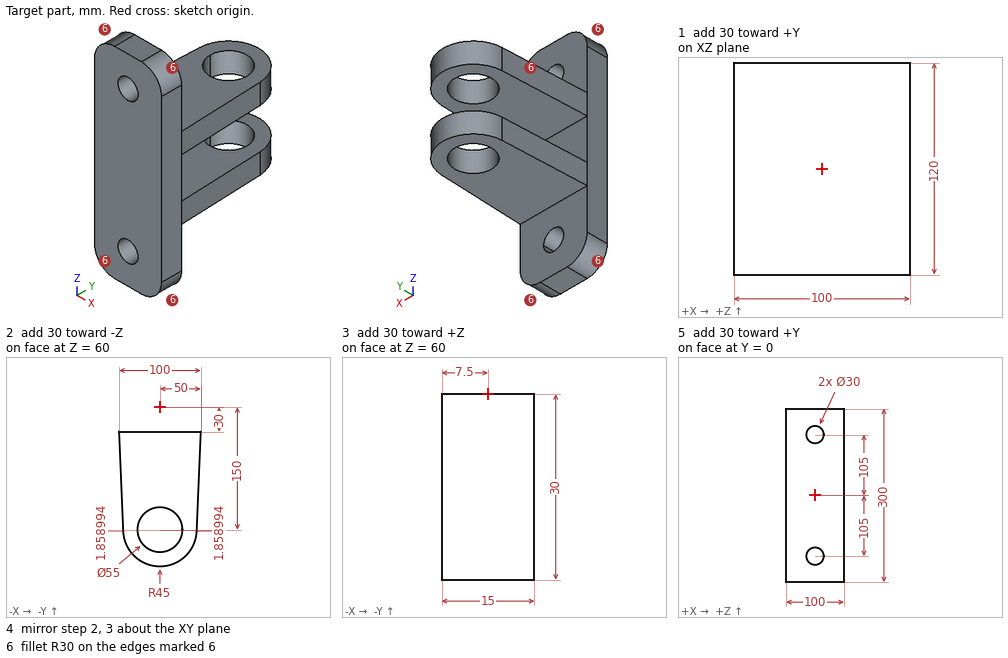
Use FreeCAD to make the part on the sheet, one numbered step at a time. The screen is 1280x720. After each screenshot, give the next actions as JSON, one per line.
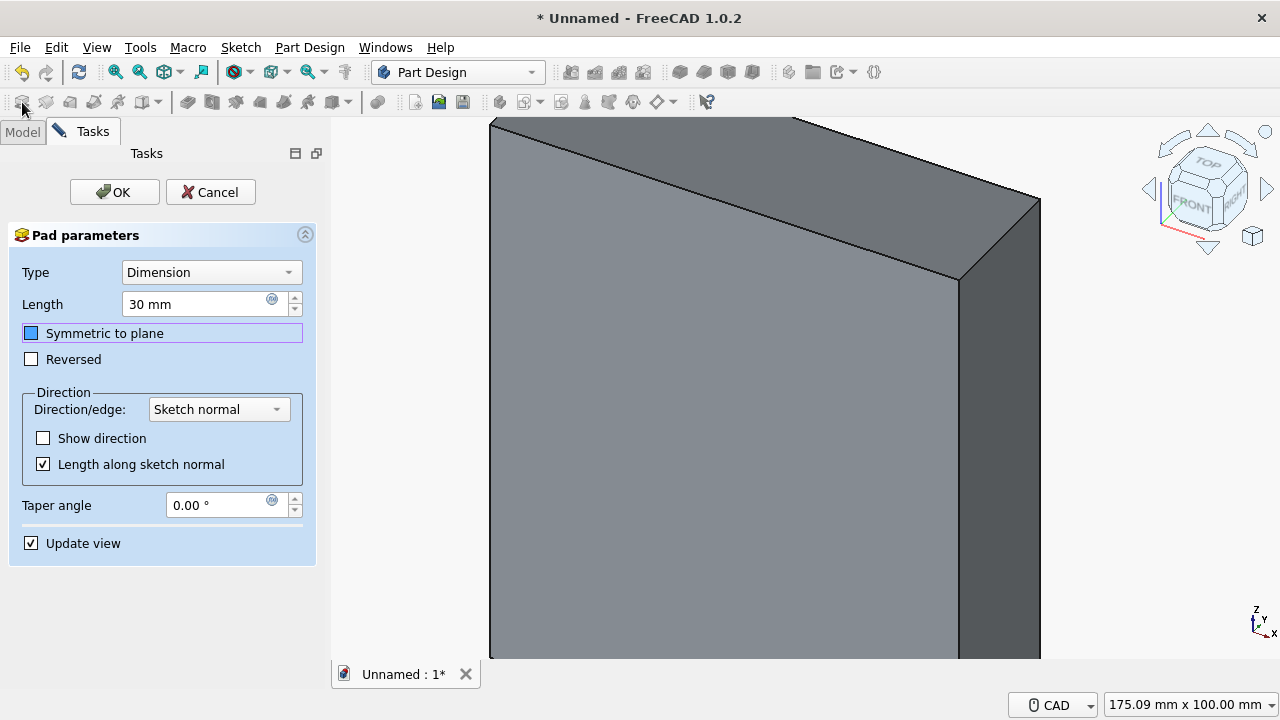
{"action": "left_click", "coordinate": [30, 359]}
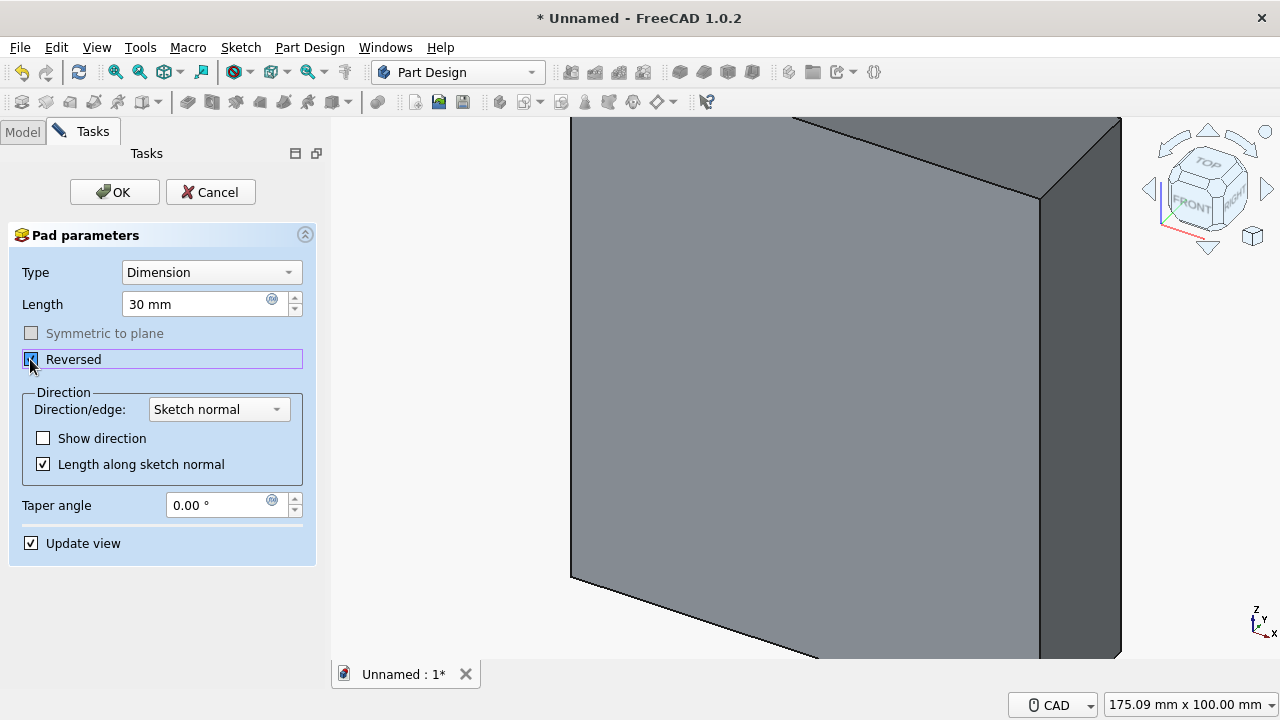
{"action": "left_click", "coordinate": [115, 192]}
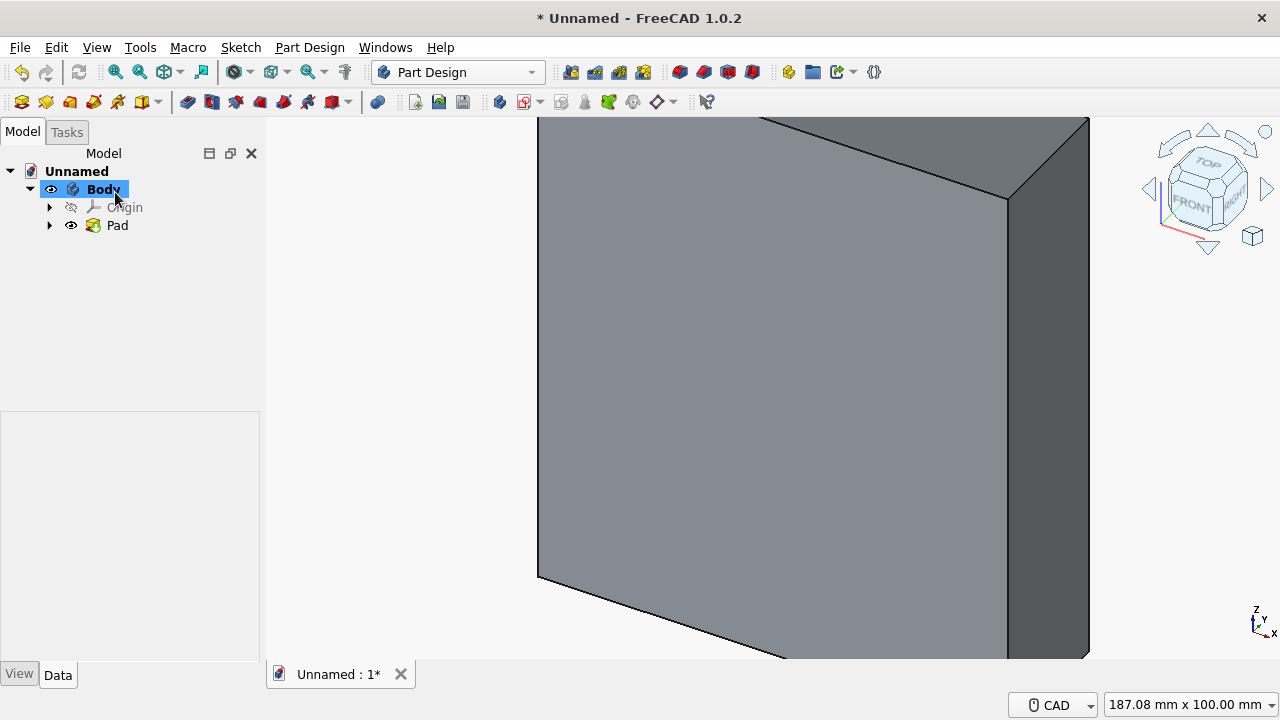
{"action": "key", "text": "v f"}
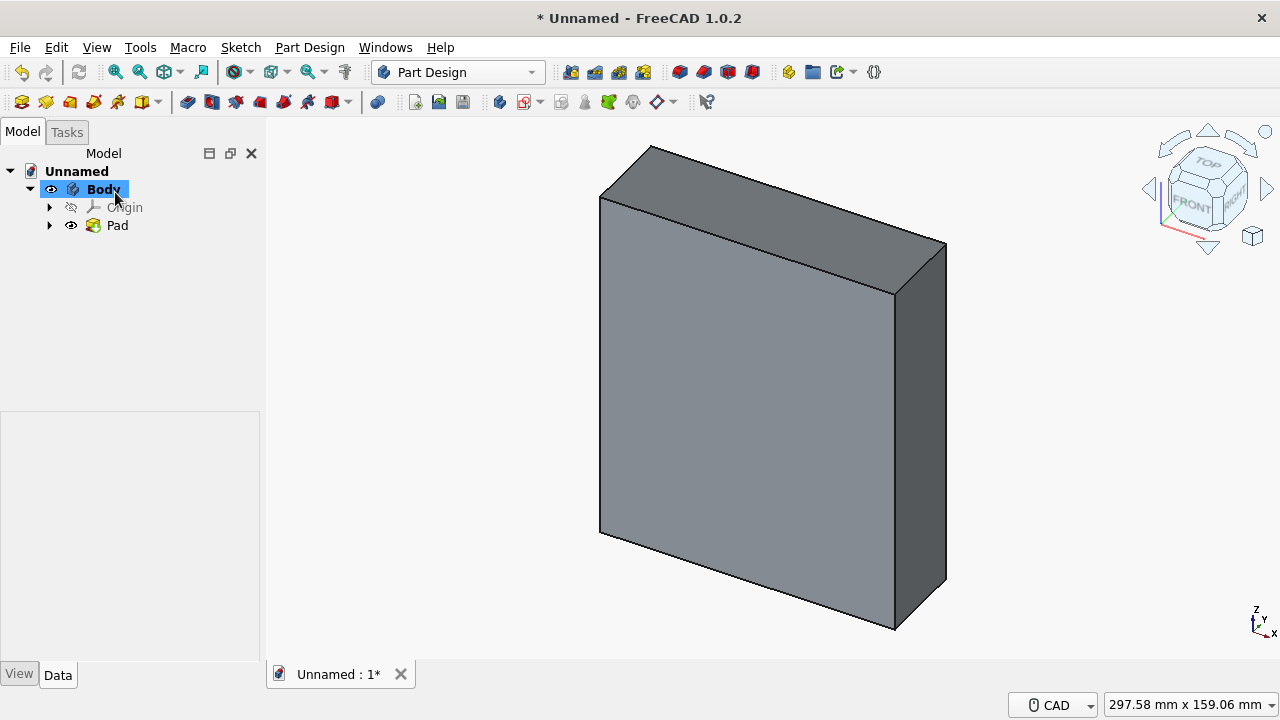
{"action": "left_click", "coordinate": [857, 247]}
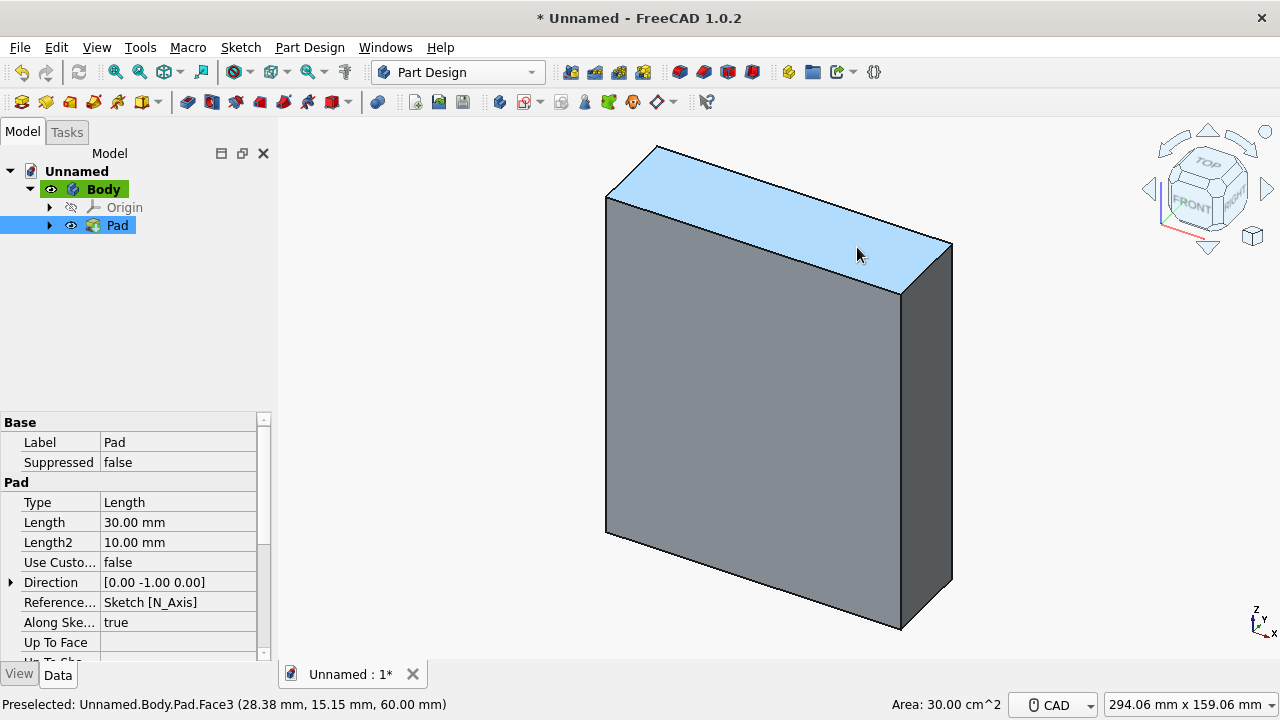
{"action": "left_click", "coordinate": [524, 102]}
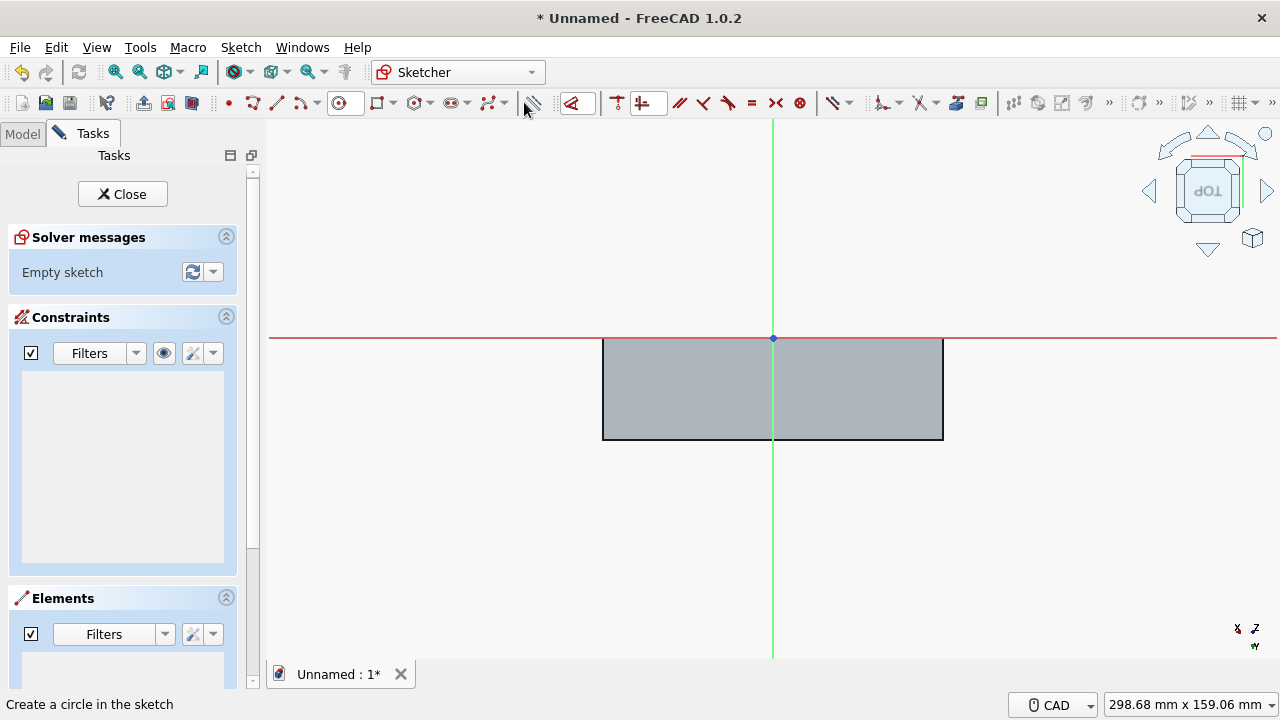
{"action": "scroll", "coordinate": [649, 160], "scroll_direction": "down", "scroll_amount": 4}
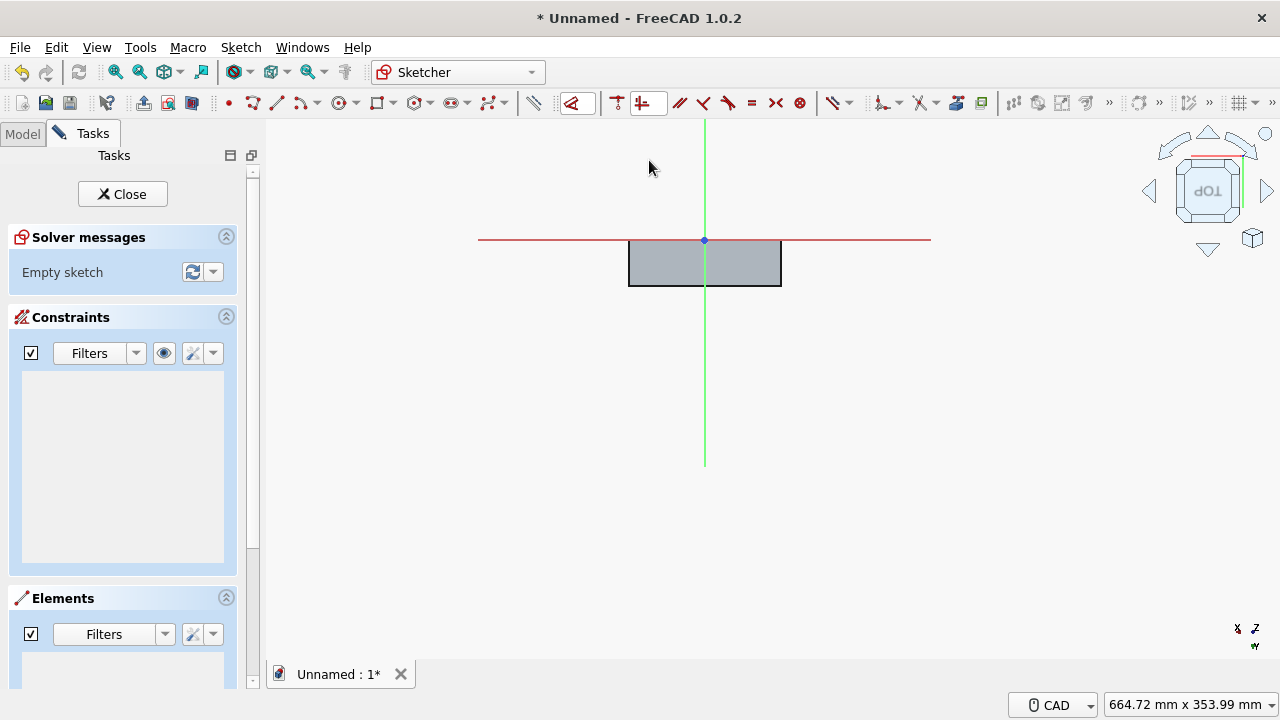
{"action": "key", "text": "g m"}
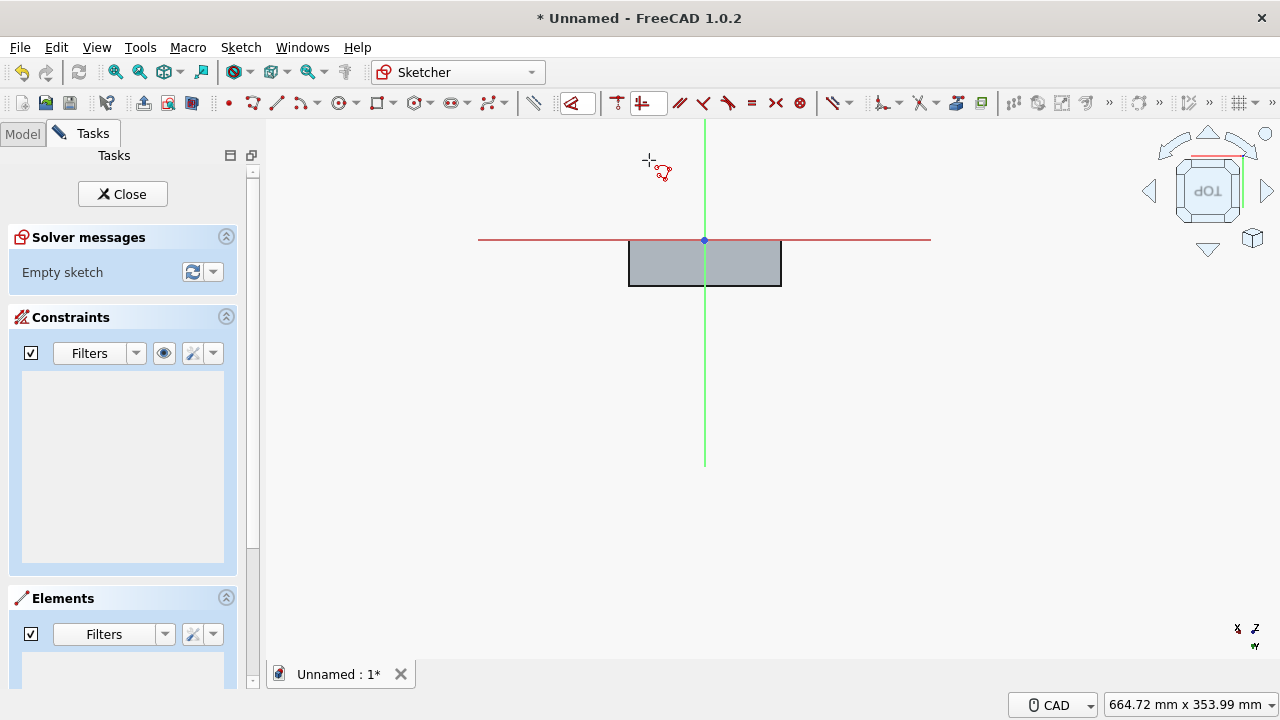
{"action": "left_click", "coordinate": [774, 472]}
{"action": "left_click", "coordinate": [784, 286]}
{"action": "left_click", "coordinate": [629, 286]}
{"action": "left_click", "coordinate": [639, 472]}
{"action": "right_click", "coordinate": [639, 472]}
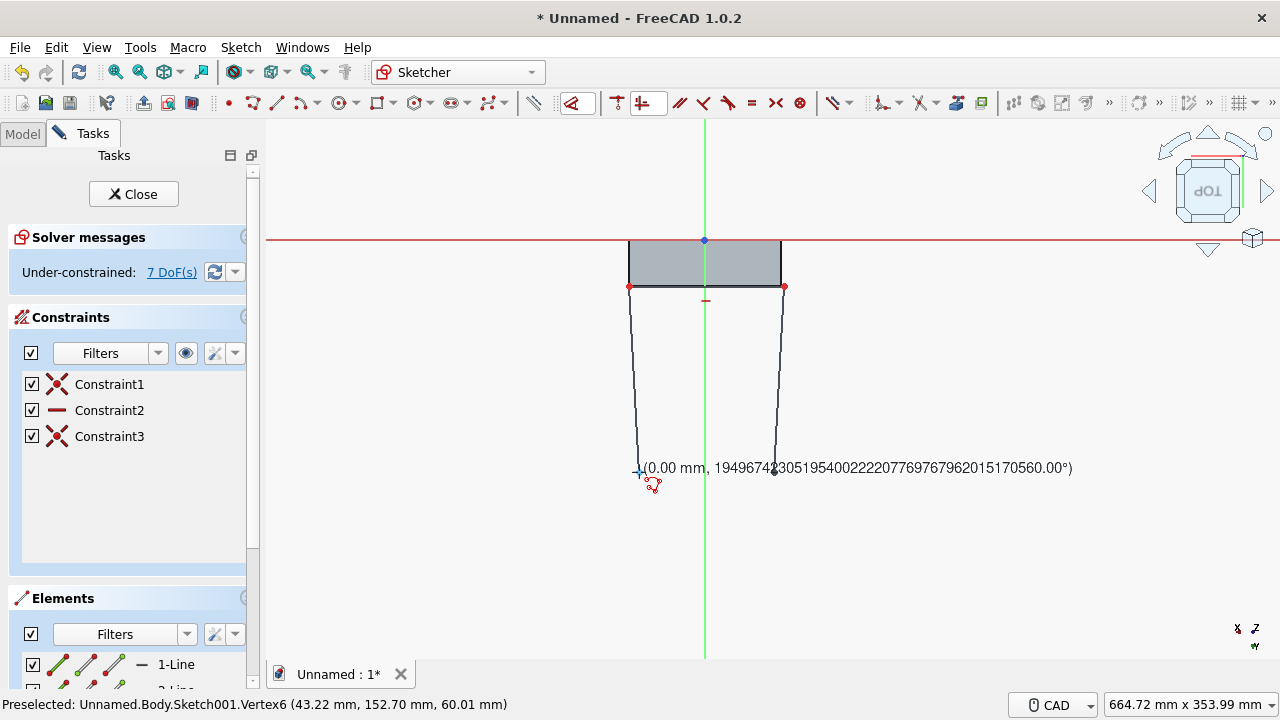
{"action": "key", "text": "g 3 a"}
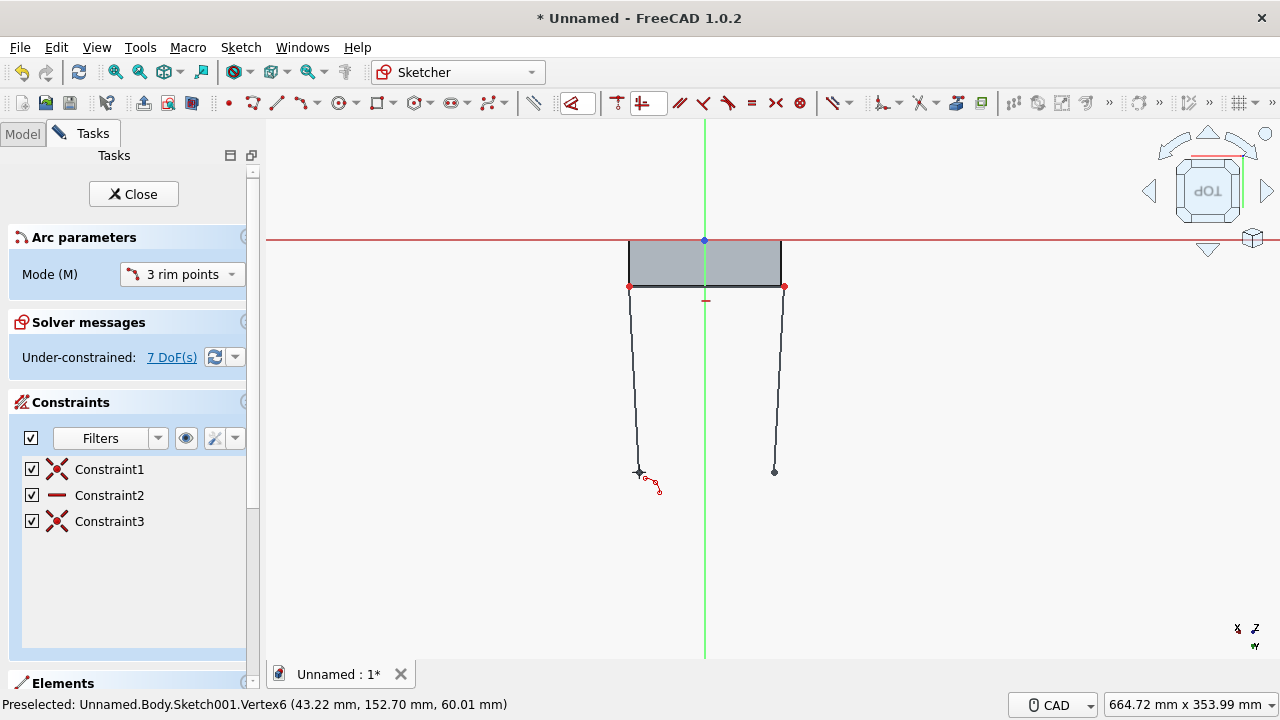
{"action": "left_click", "coordinate": [639, 473]}
{"action": "left_click", "coordinate": [774, 473]}
{"action": "left_click", "coordinate": [684, 534]}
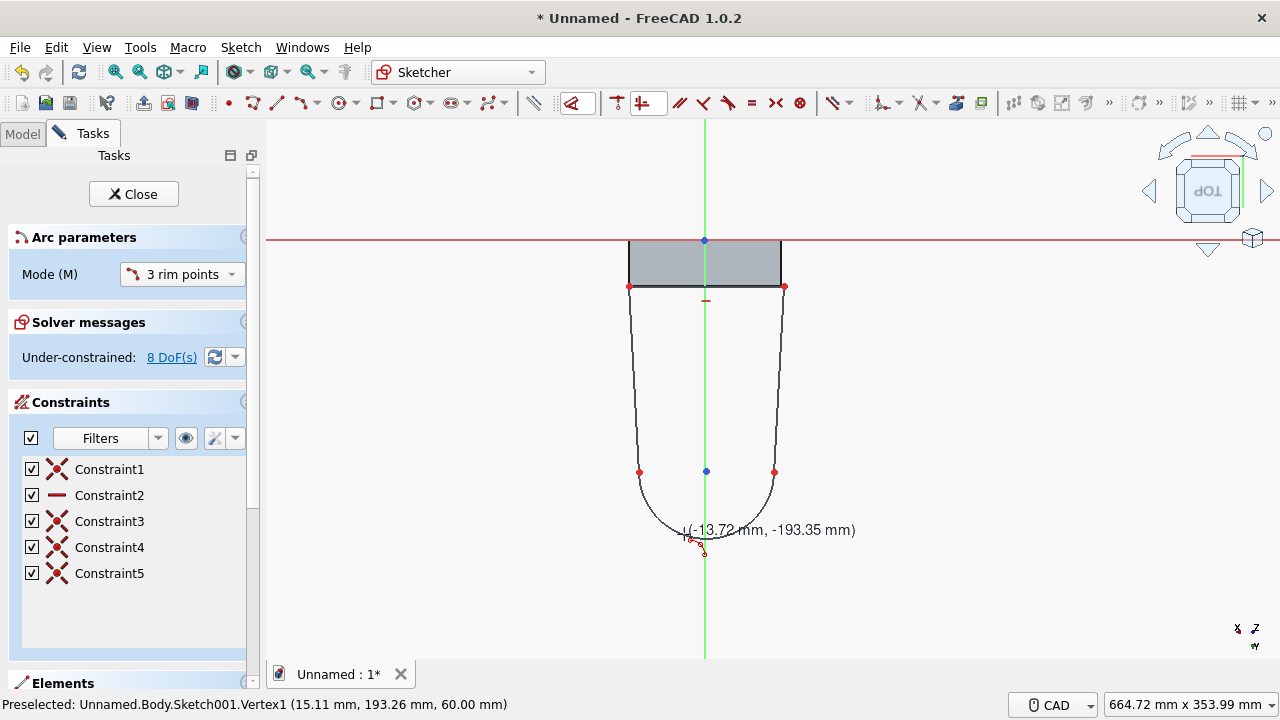
{"action": "key", "text": "g c"}